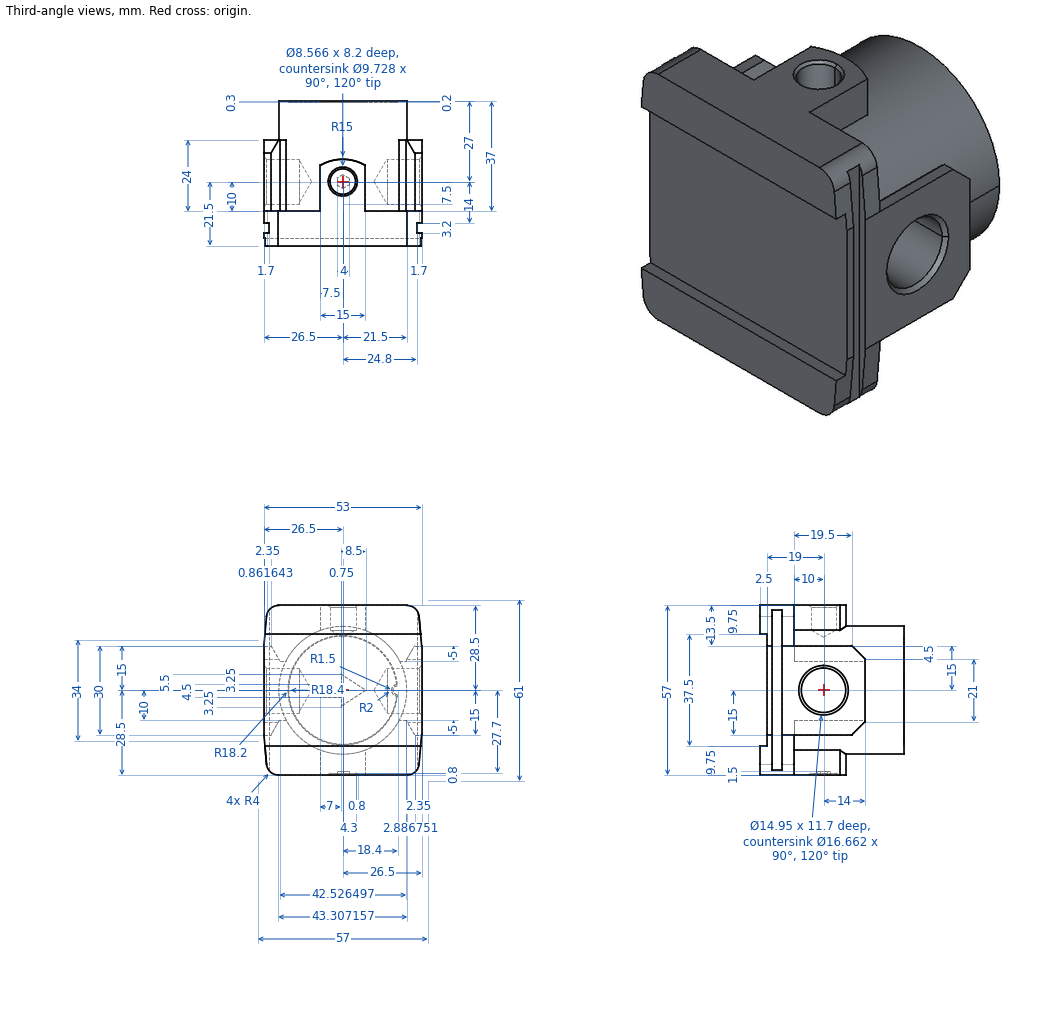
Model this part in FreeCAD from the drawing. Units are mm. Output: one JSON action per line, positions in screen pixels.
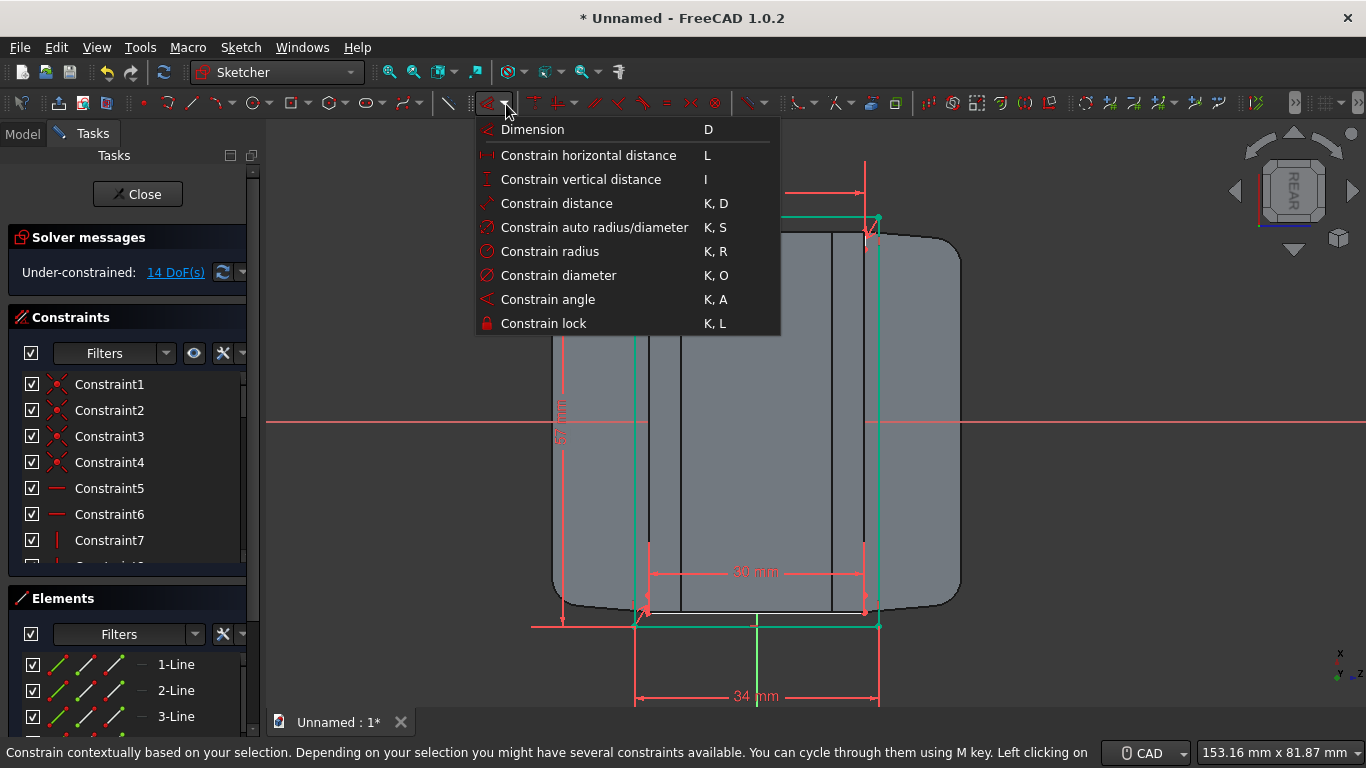
{"action": "left_click", "coordinate": [628, 155]}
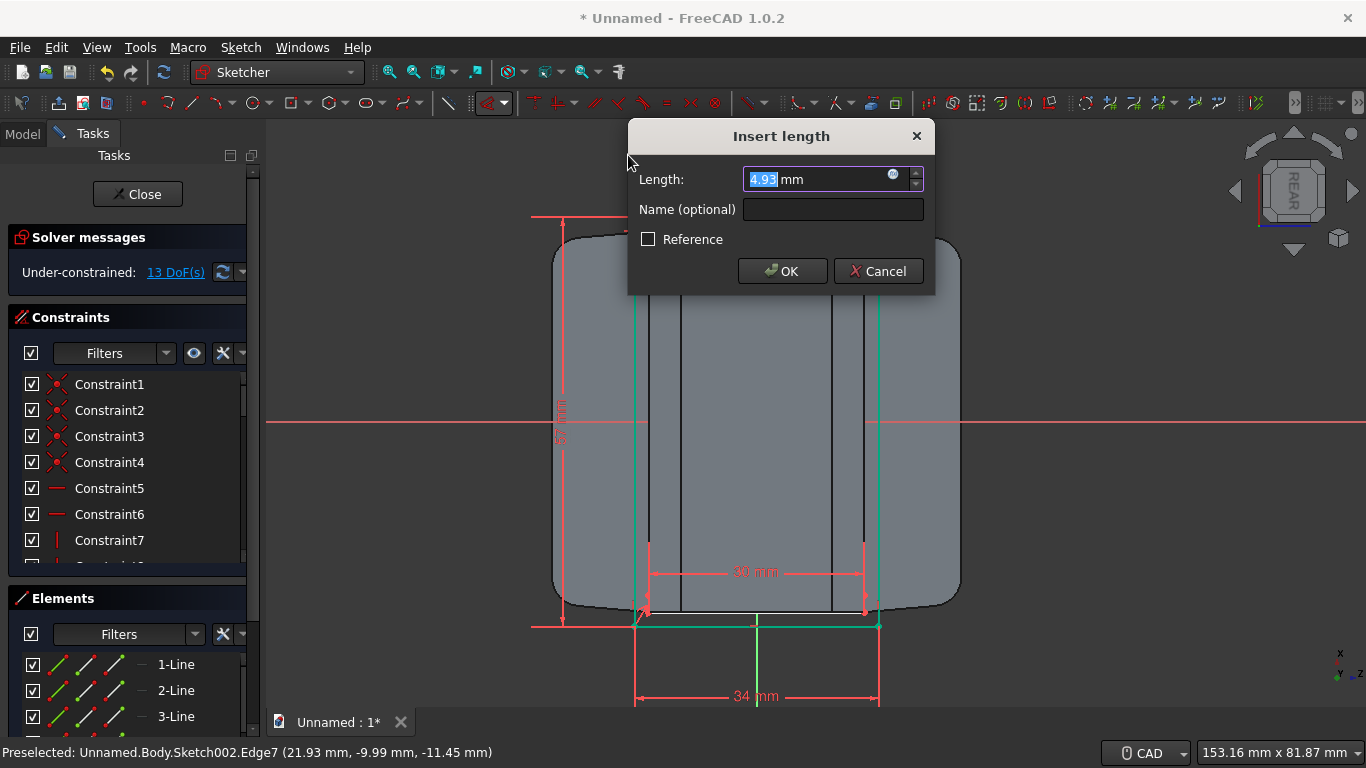
{"action": "type", "text": "5"}
{"action": "key", "text": "Return"}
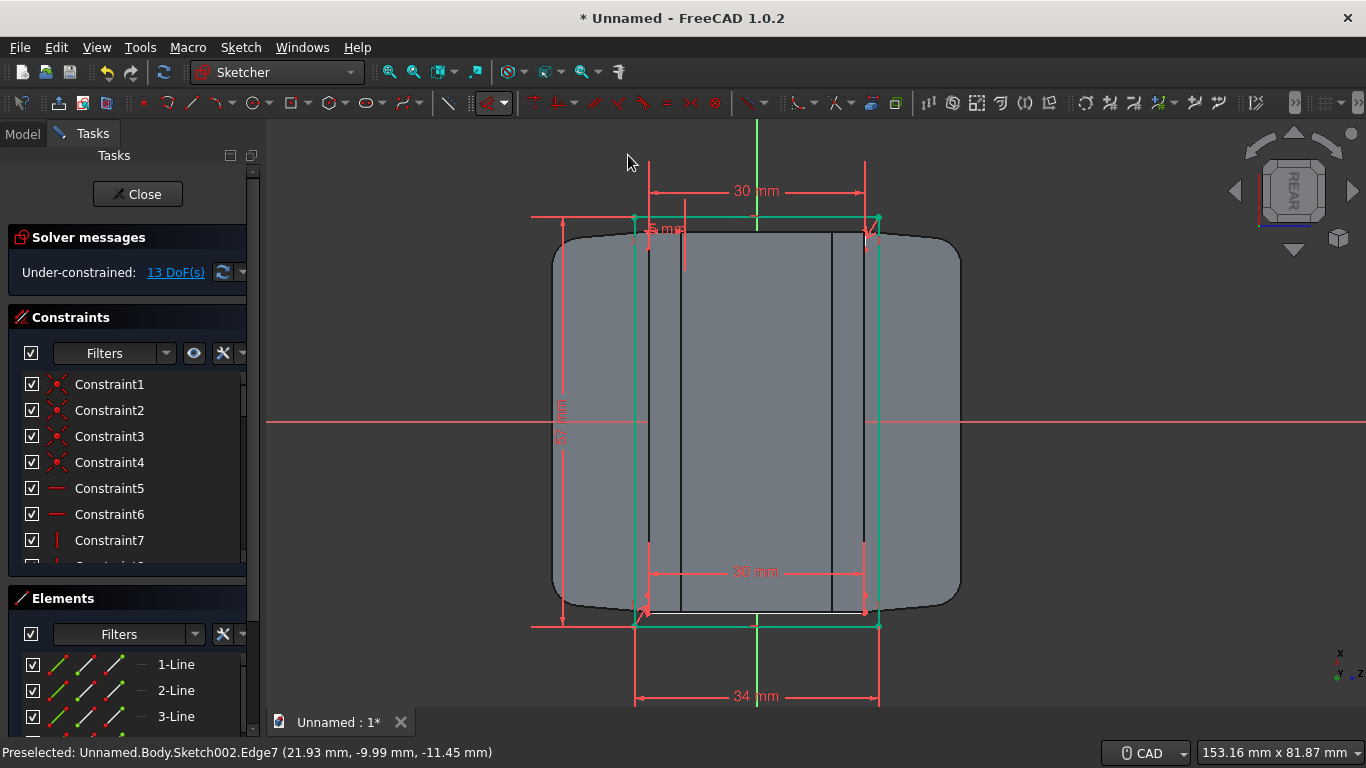
{"action": "left_click", "coordinate": [854, 255]}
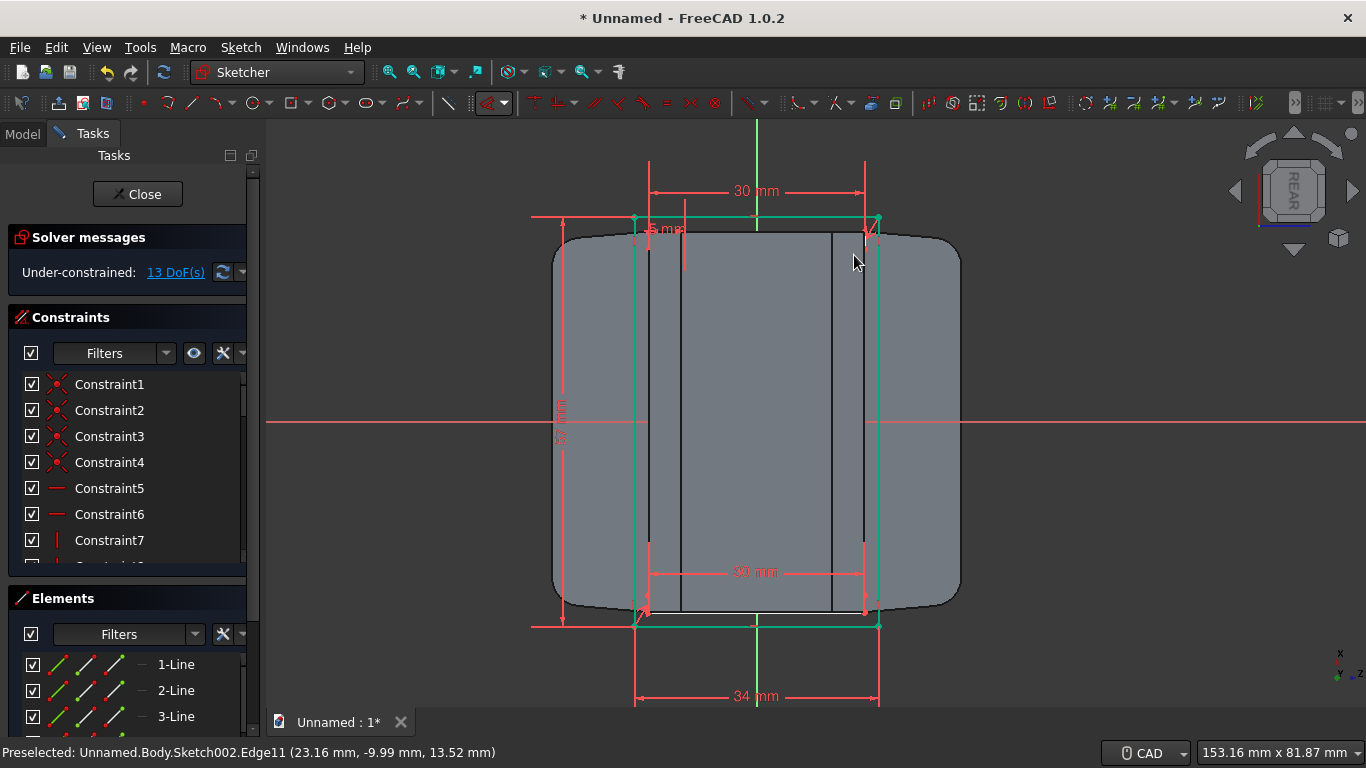
{"action": "left_click", "coordinate": [506, 104]}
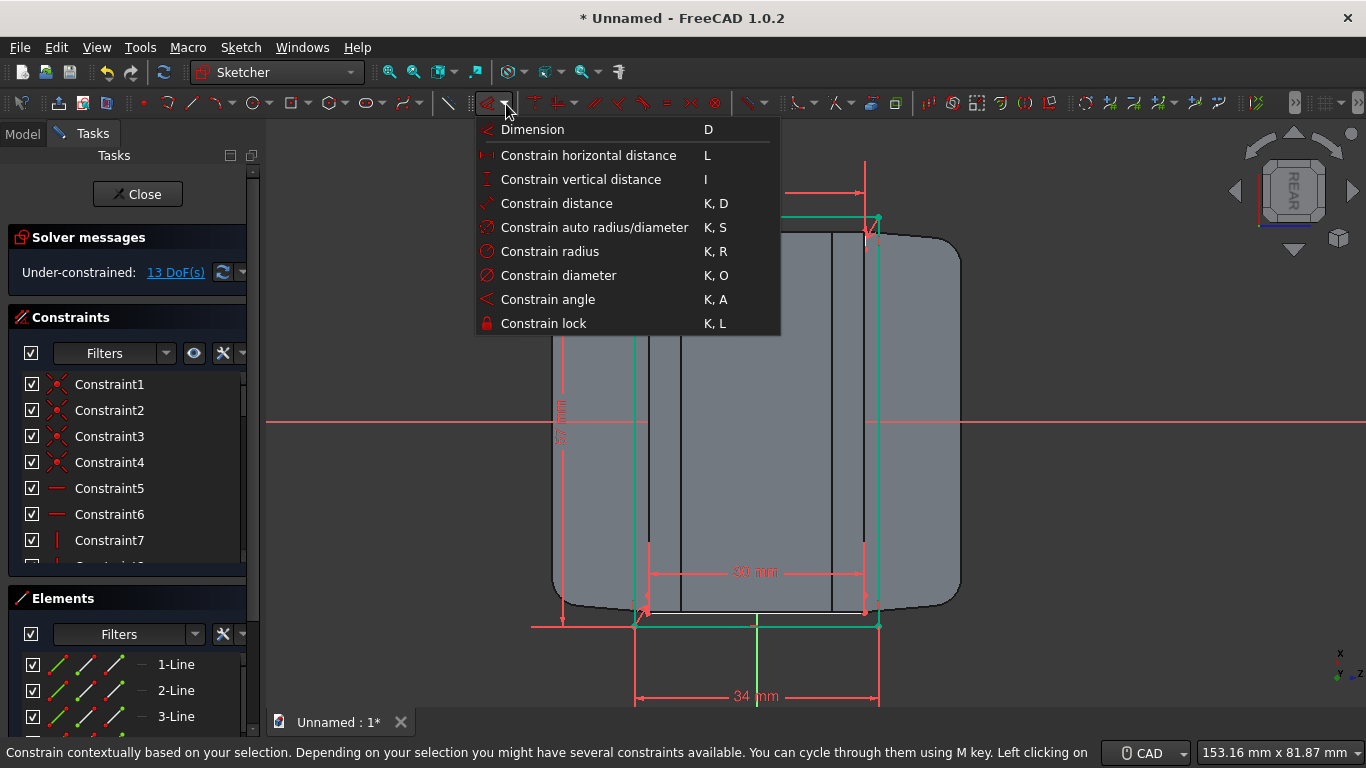
{"action": "left_click", "coordinate": [628, 155]}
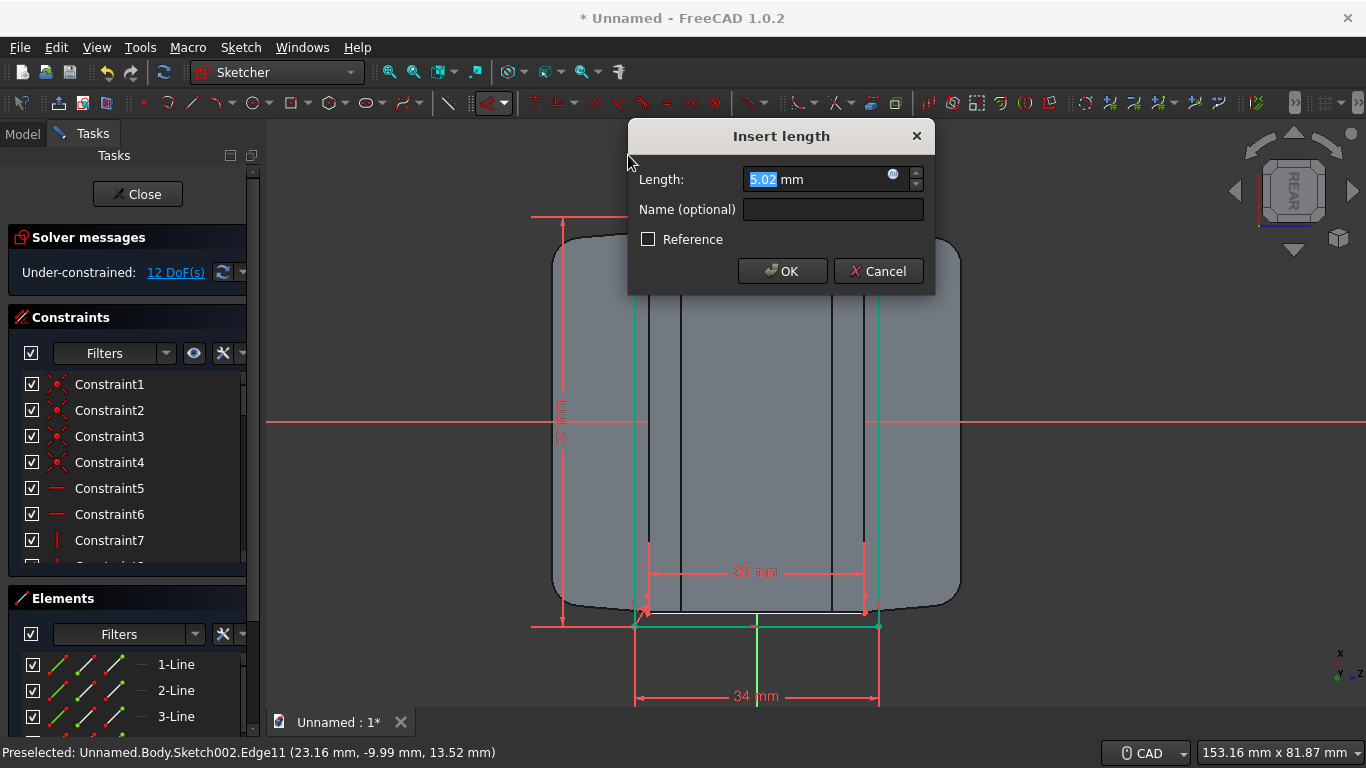
{"action": "type", "text": "5"}
{"action": "key", "text": "Return"}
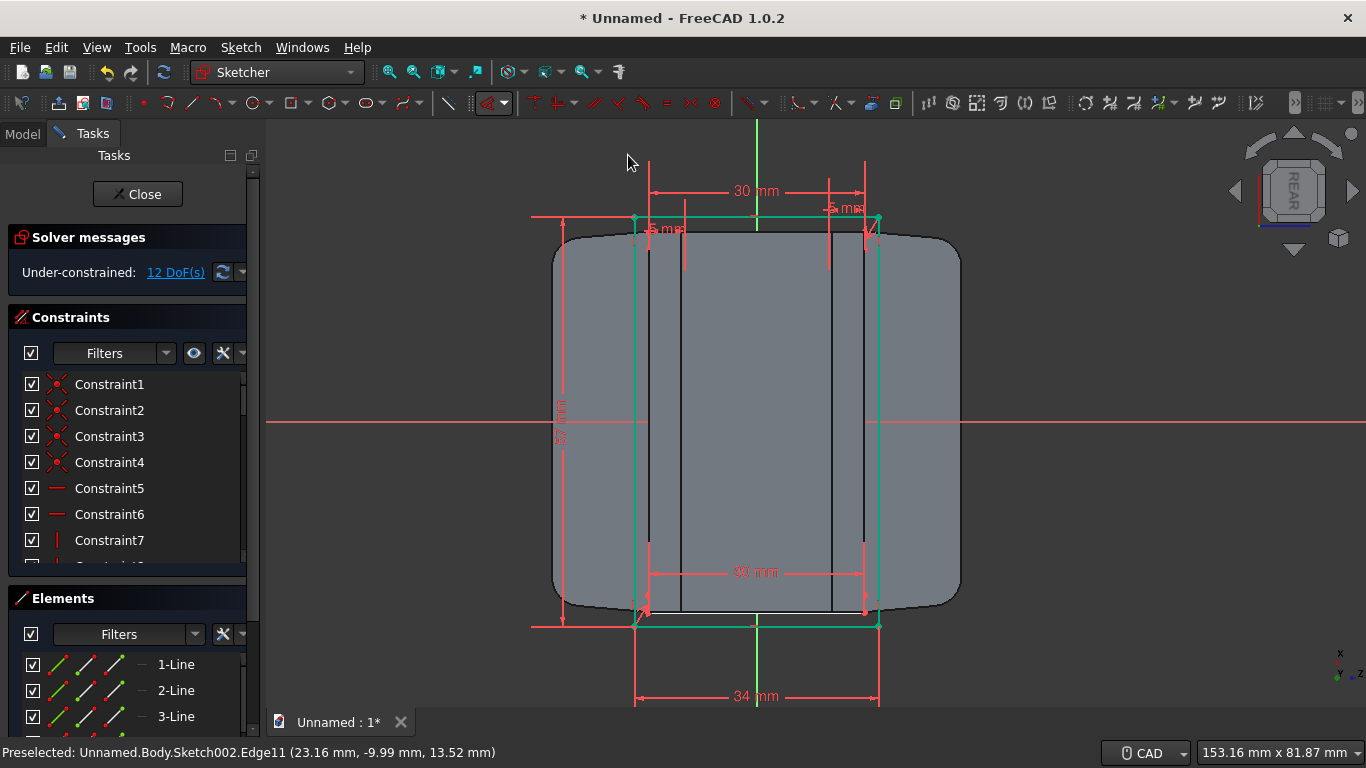
{"action": "left_click", "coordinate": [839, 581]}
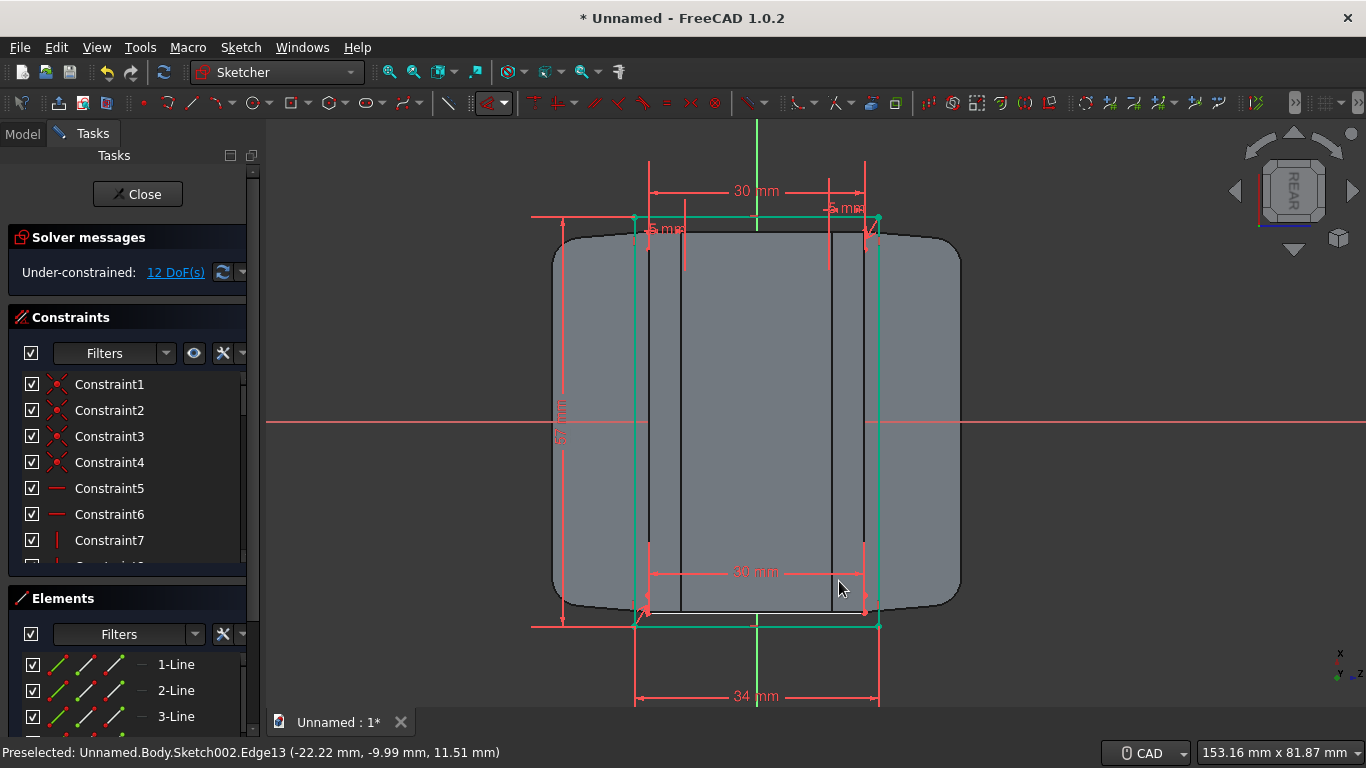
{"action": "left_click", "coordinate": [506, 104]}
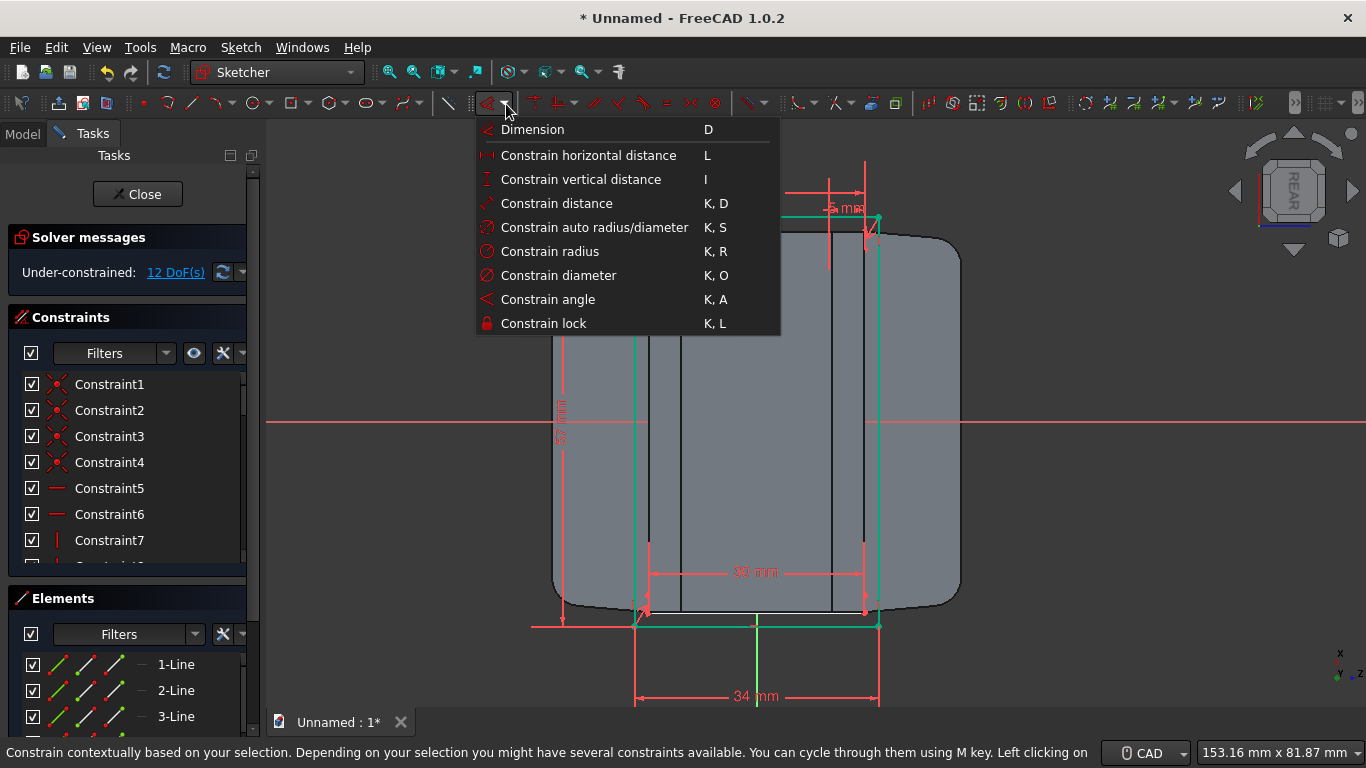
{"action": "left_click", "coordinate": [628, 155]}